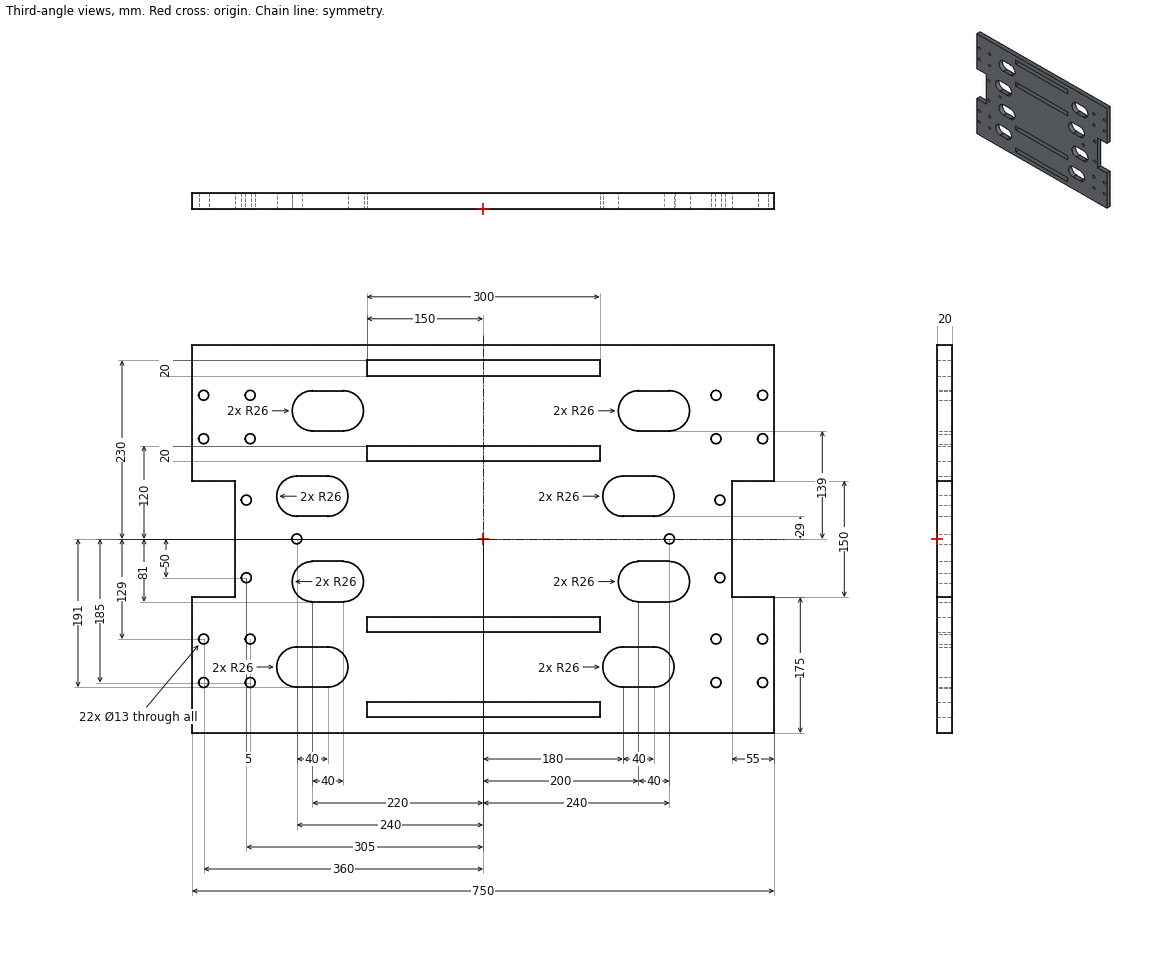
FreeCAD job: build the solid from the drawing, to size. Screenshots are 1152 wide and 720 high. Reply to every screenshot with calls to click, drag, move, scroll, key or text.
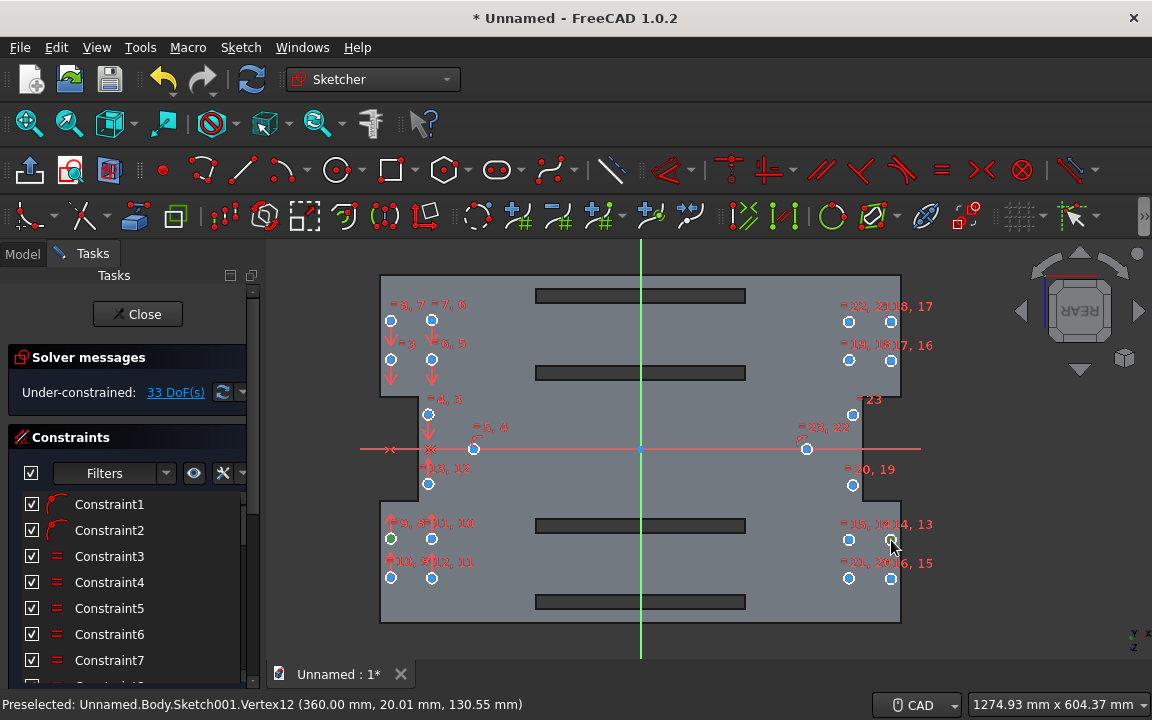
click(641, 605)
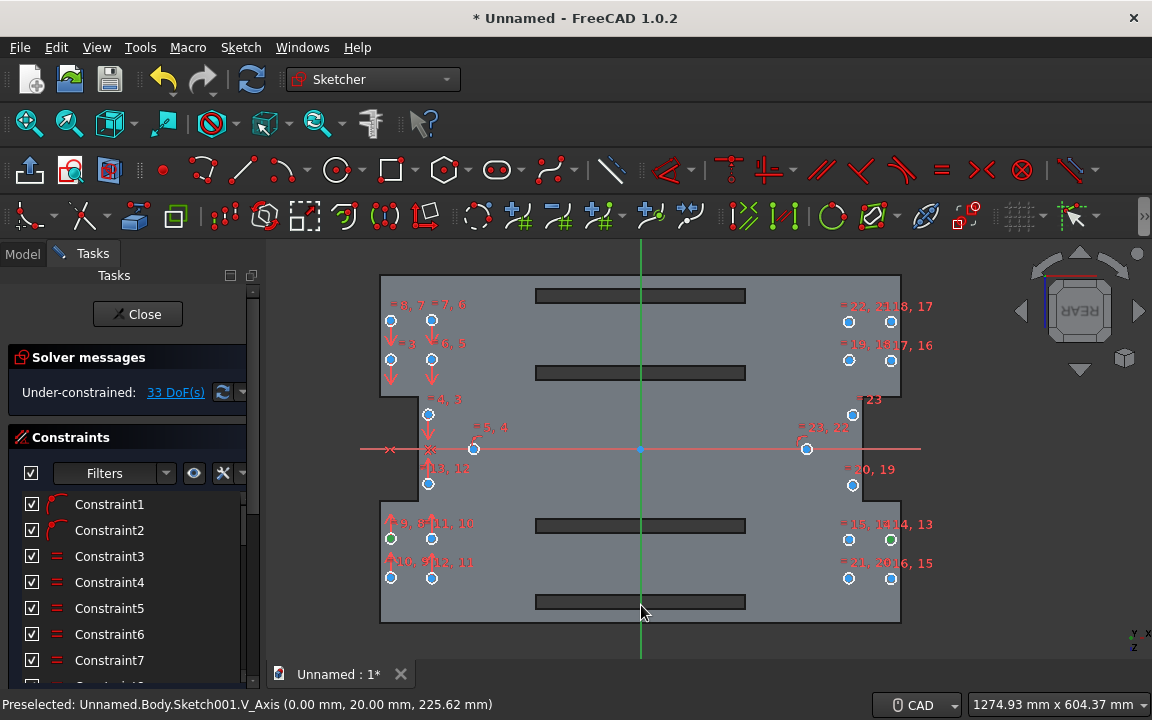
click(982, 170)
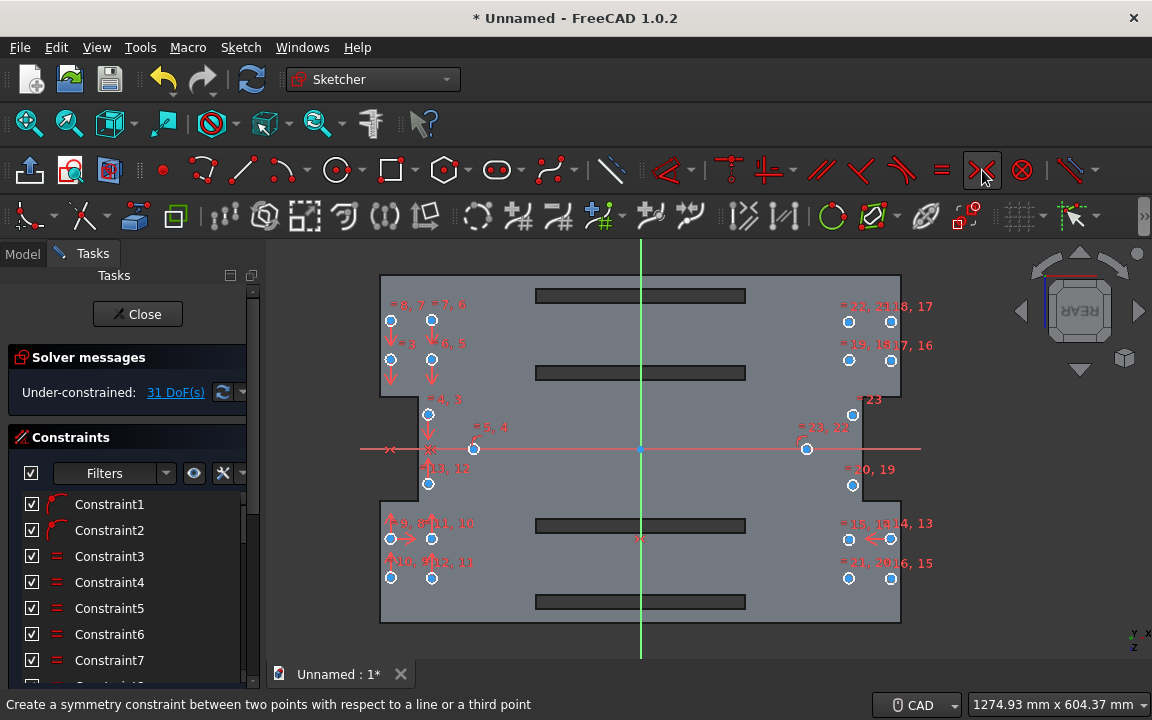
click(432, 539)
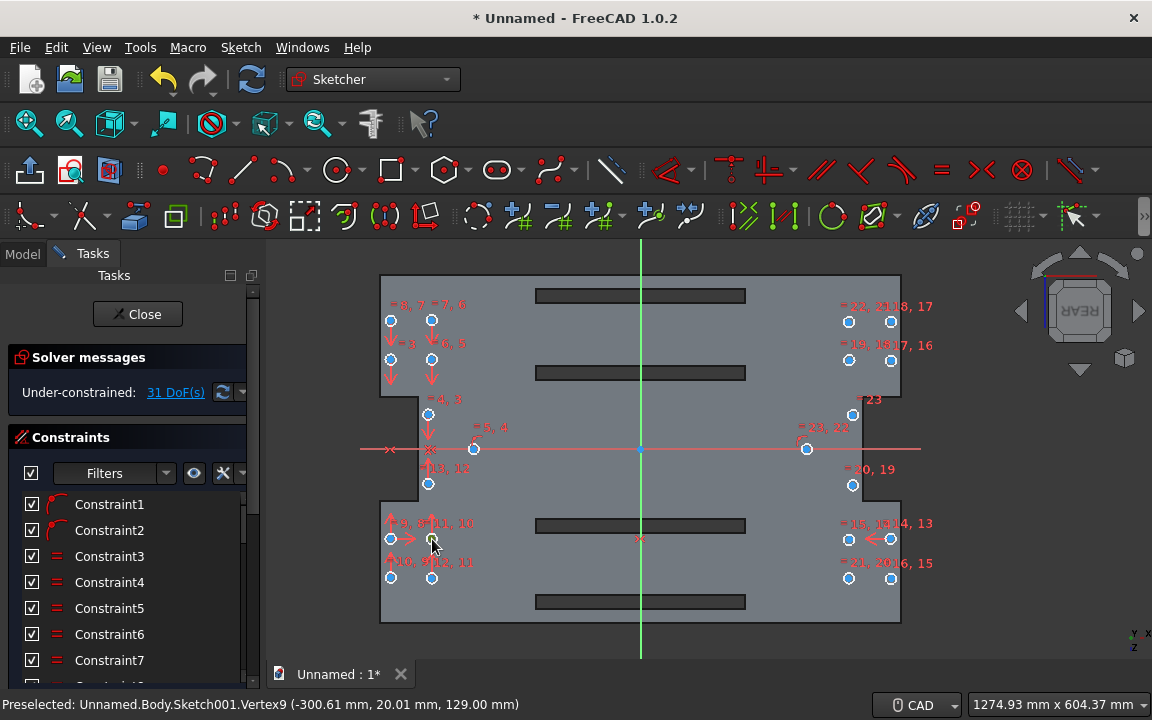
click(849, 540)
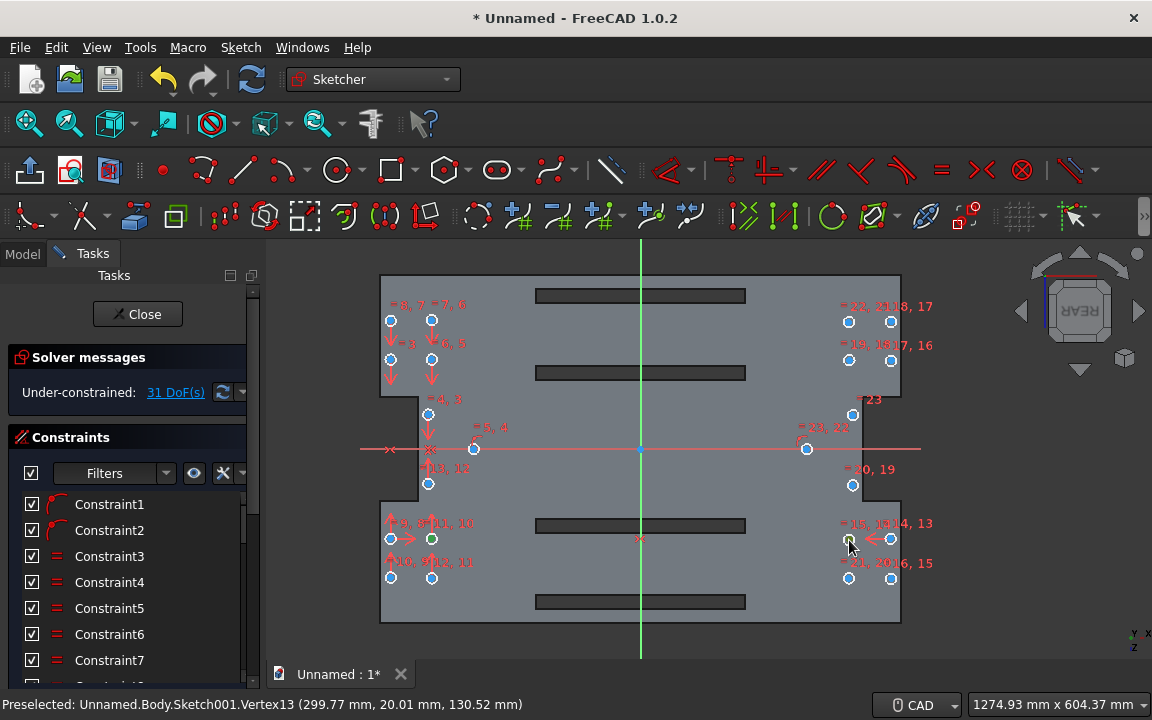
click(641, 605)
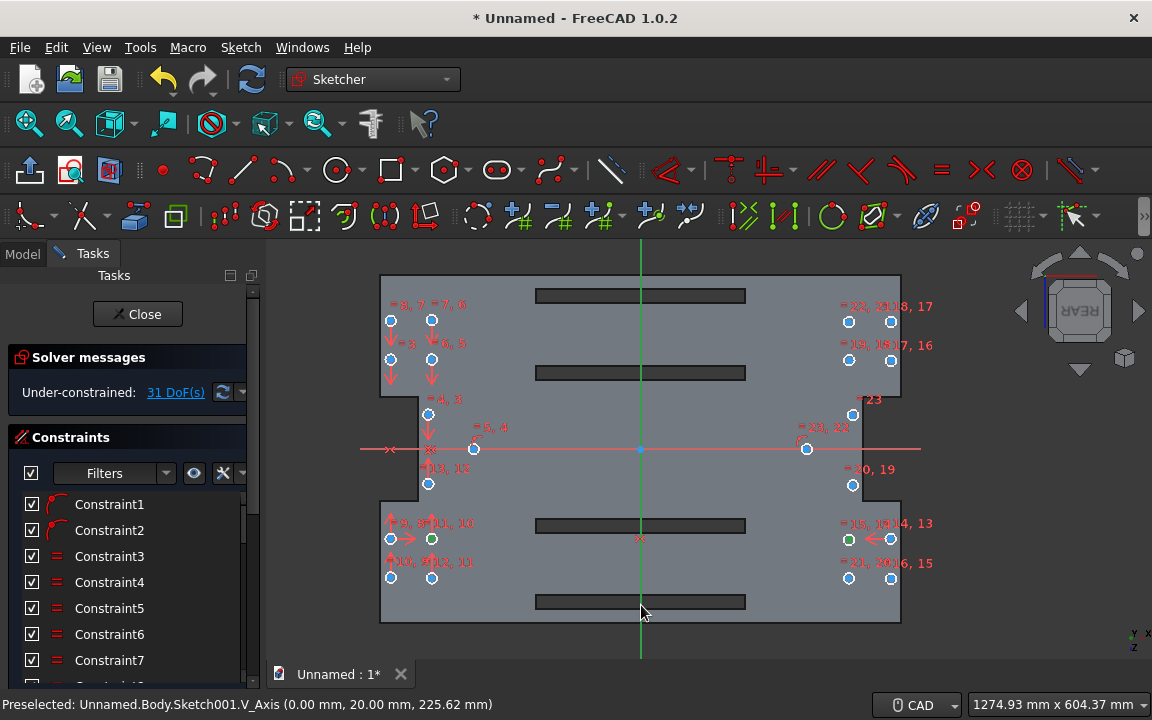
click(982, 170)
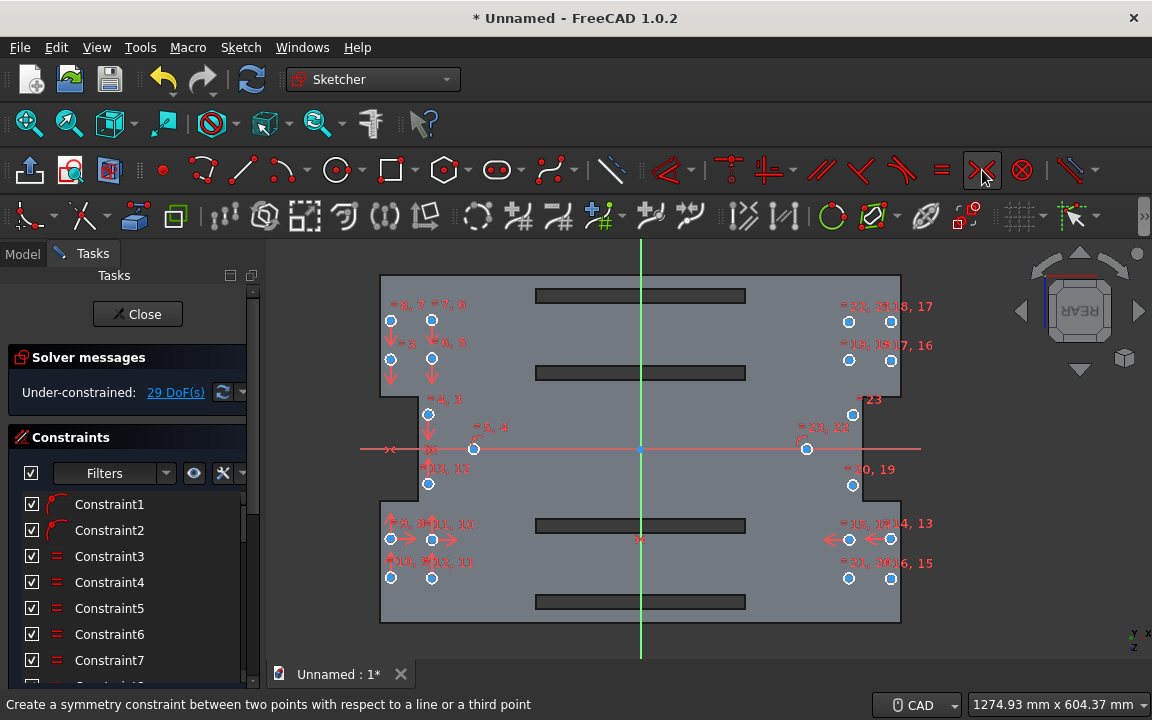
click(391, 578)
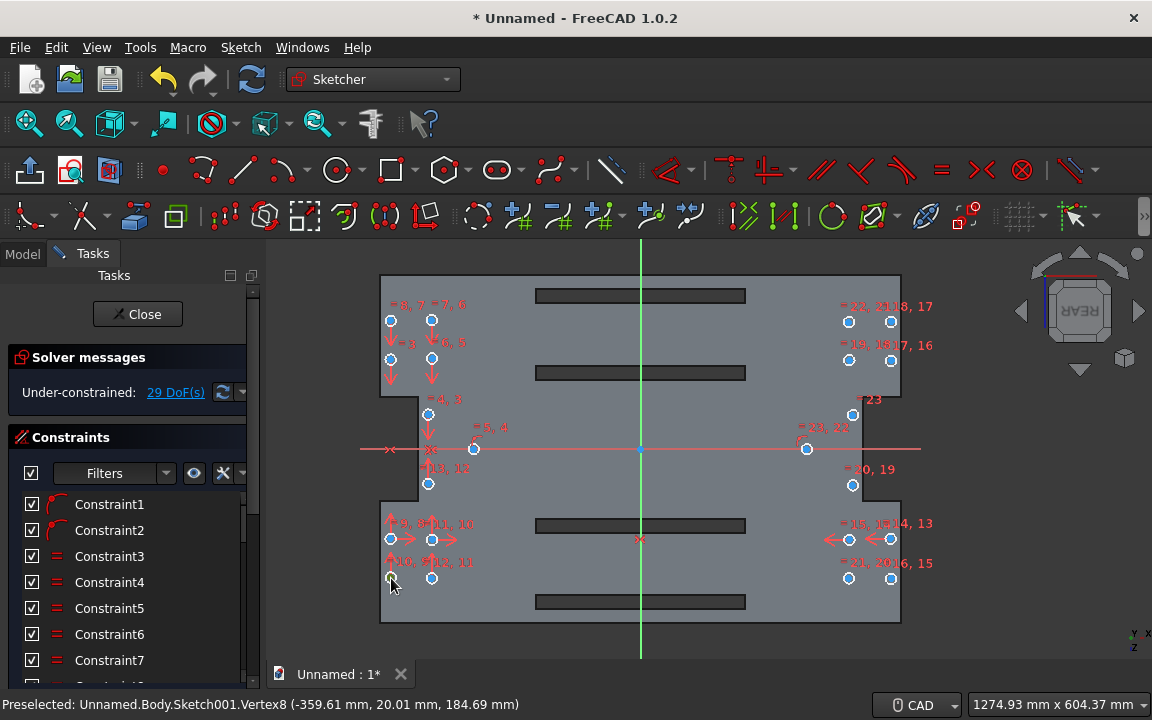
click(891, 579)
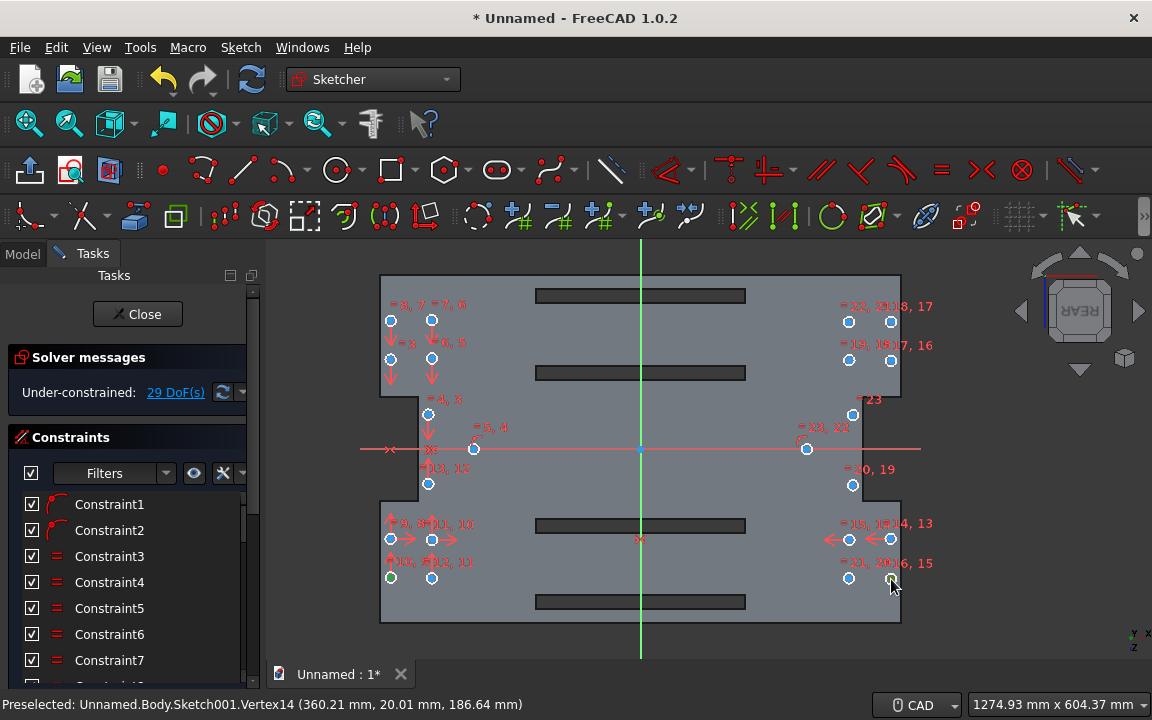
click(641, 605)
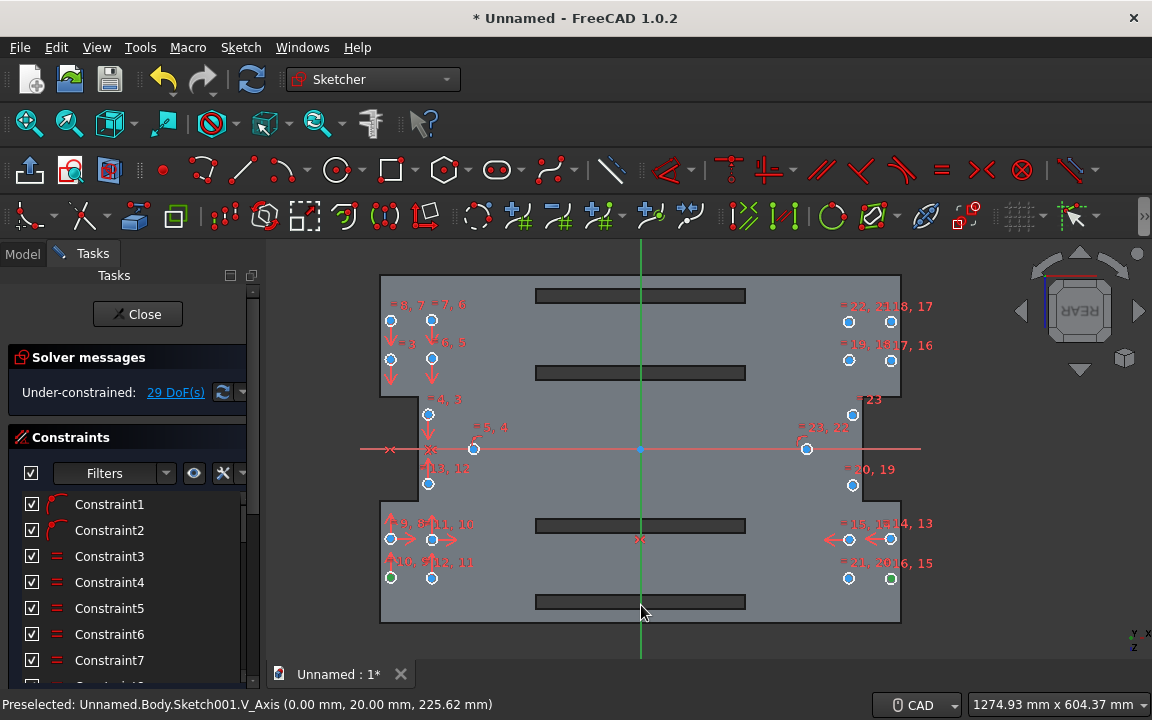
click(982, 170)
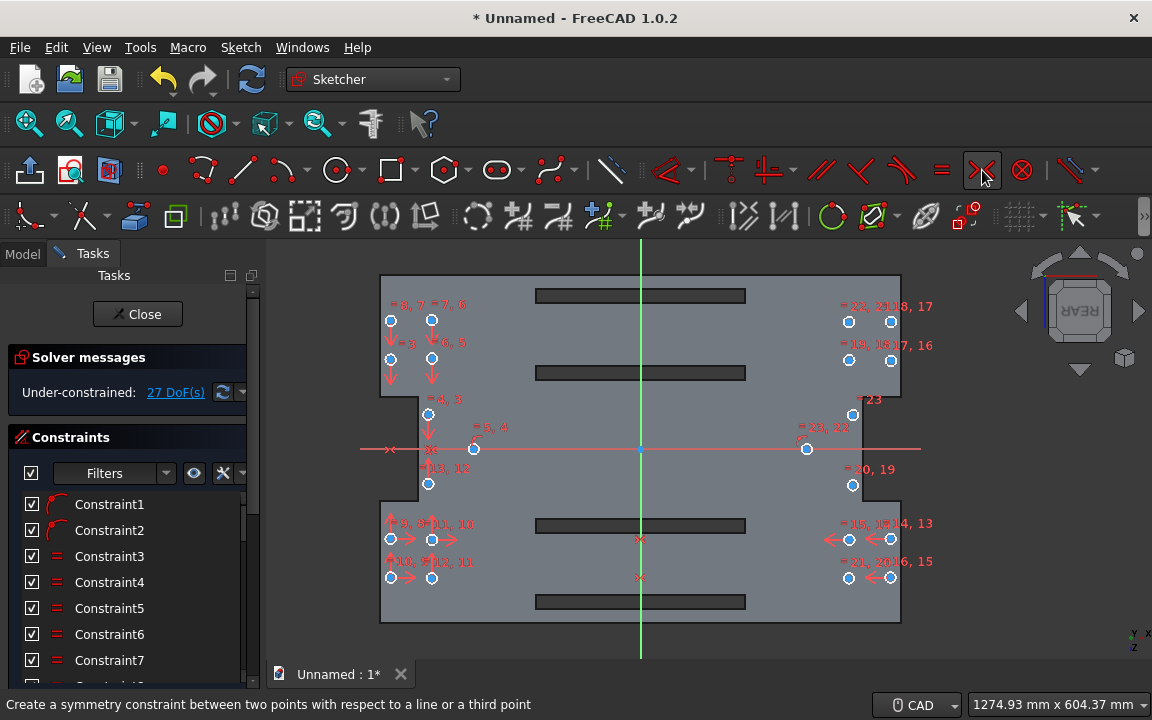
click(391, 360)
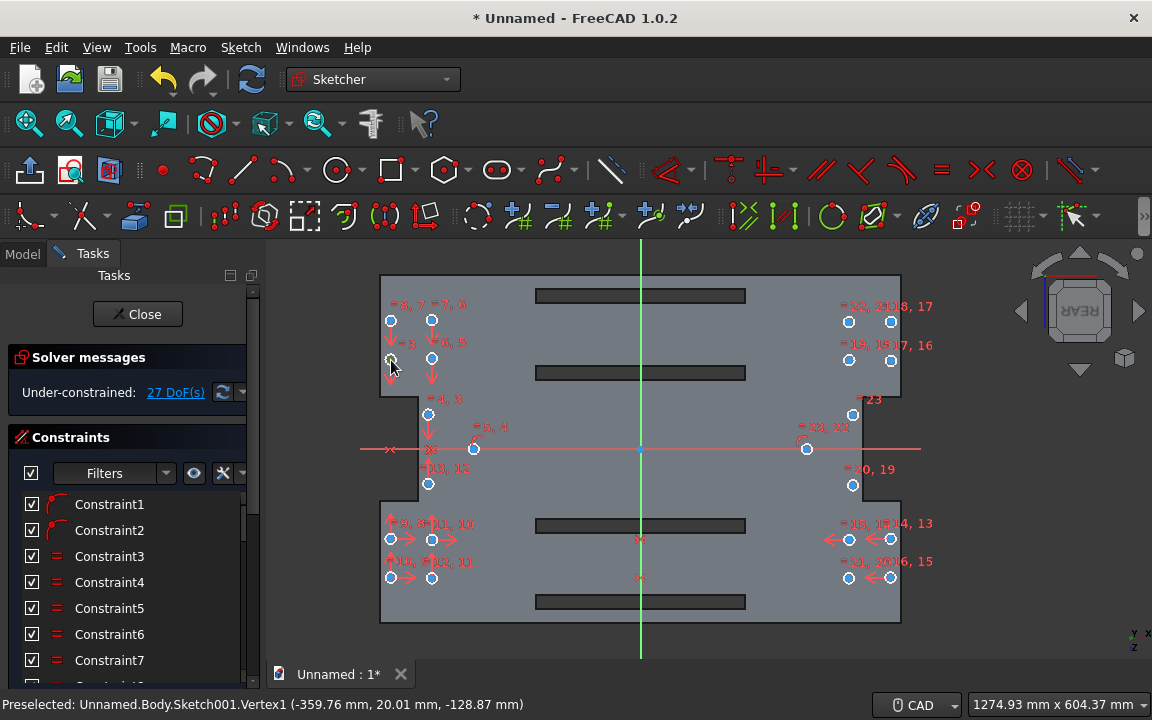
click(891, 361)